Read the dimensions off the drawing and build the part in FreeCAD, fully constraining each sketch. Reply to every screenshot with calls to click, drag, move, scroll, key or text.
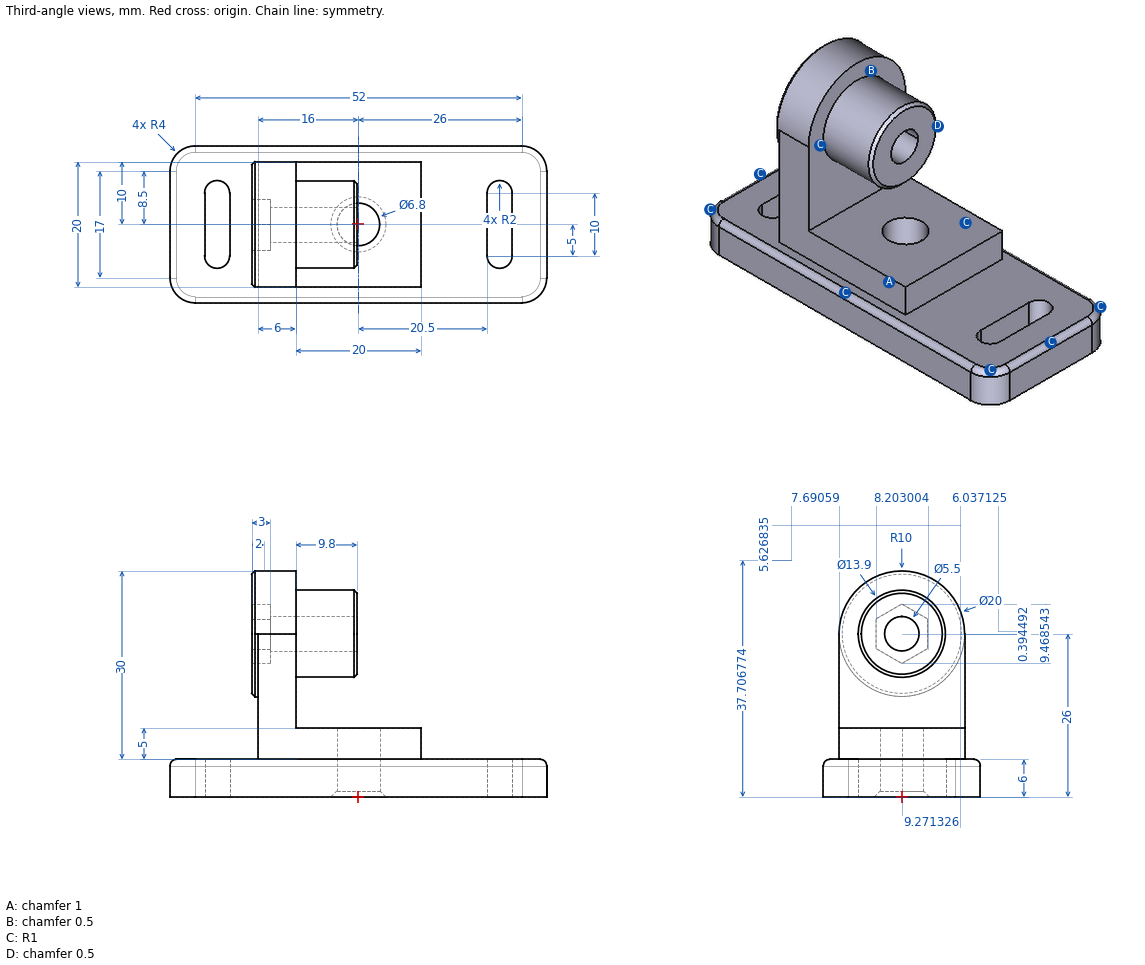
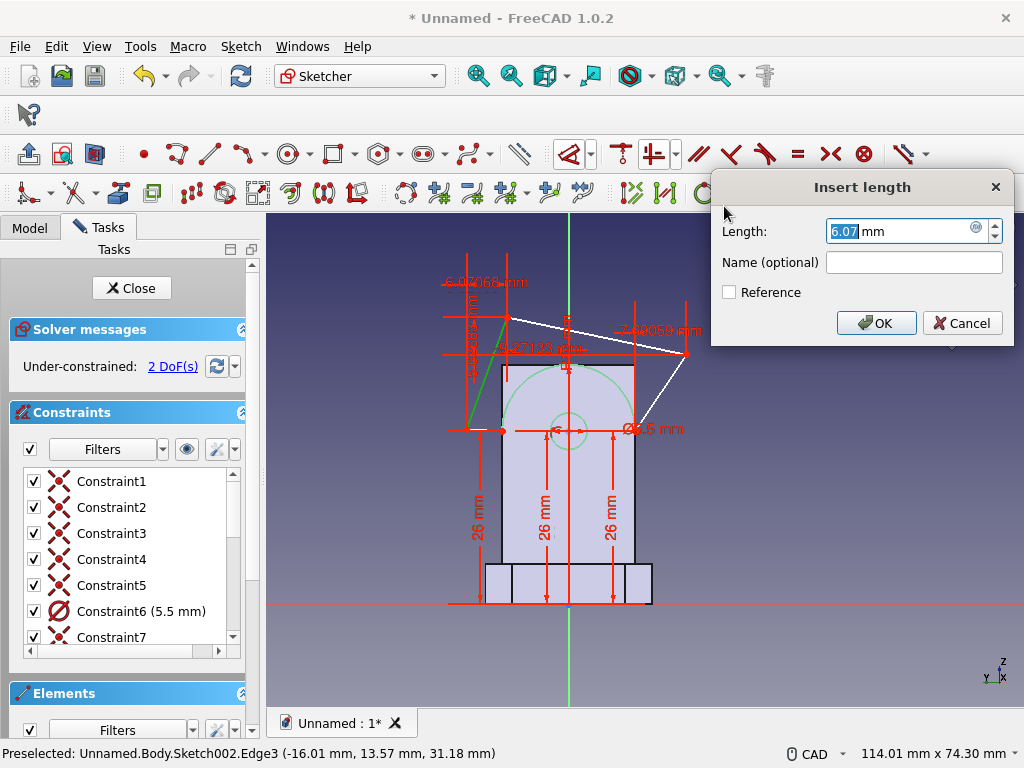
text(6.037125)
key(Return)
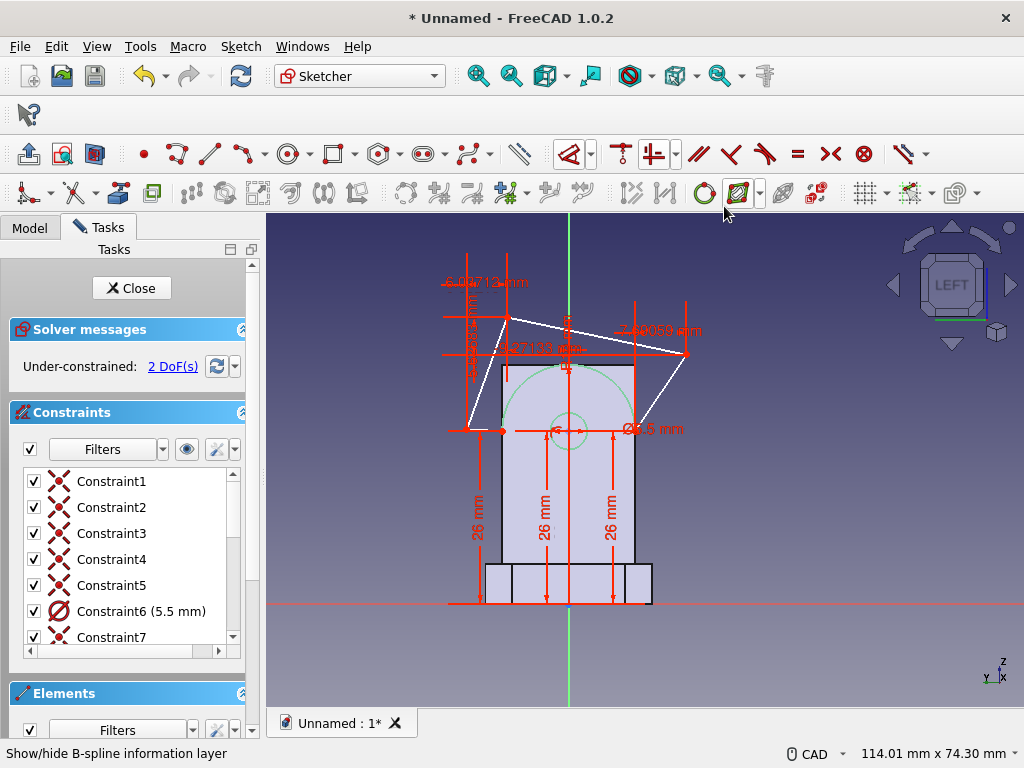
scroll(478, 430, up, 14)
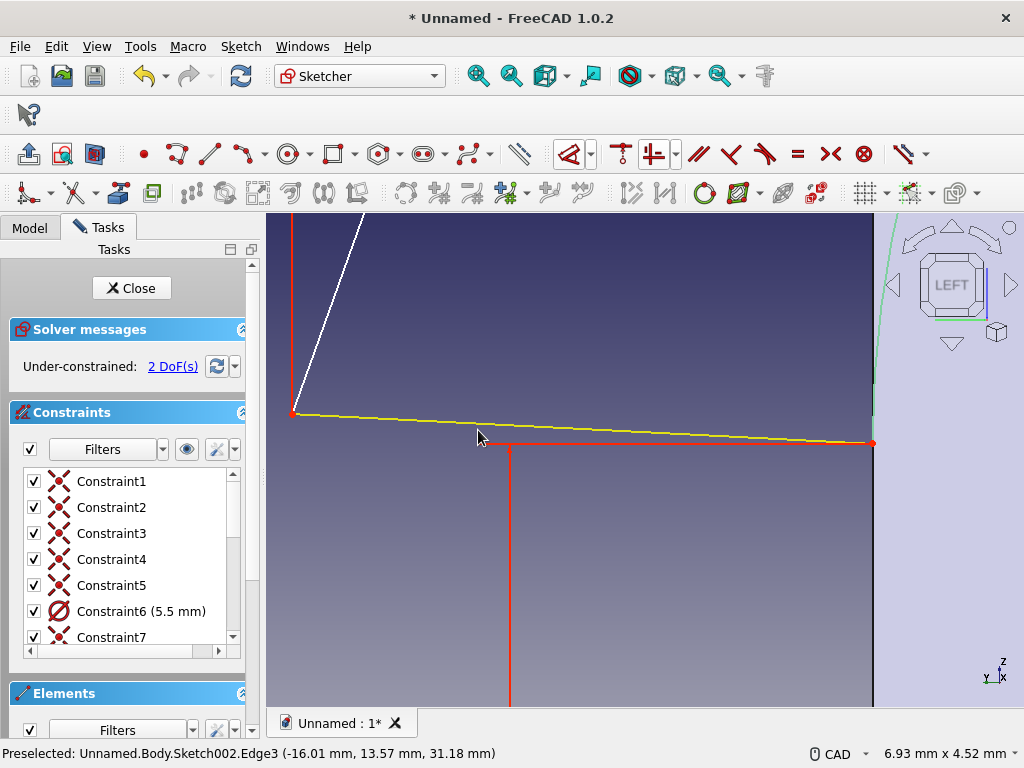
click(466, 423)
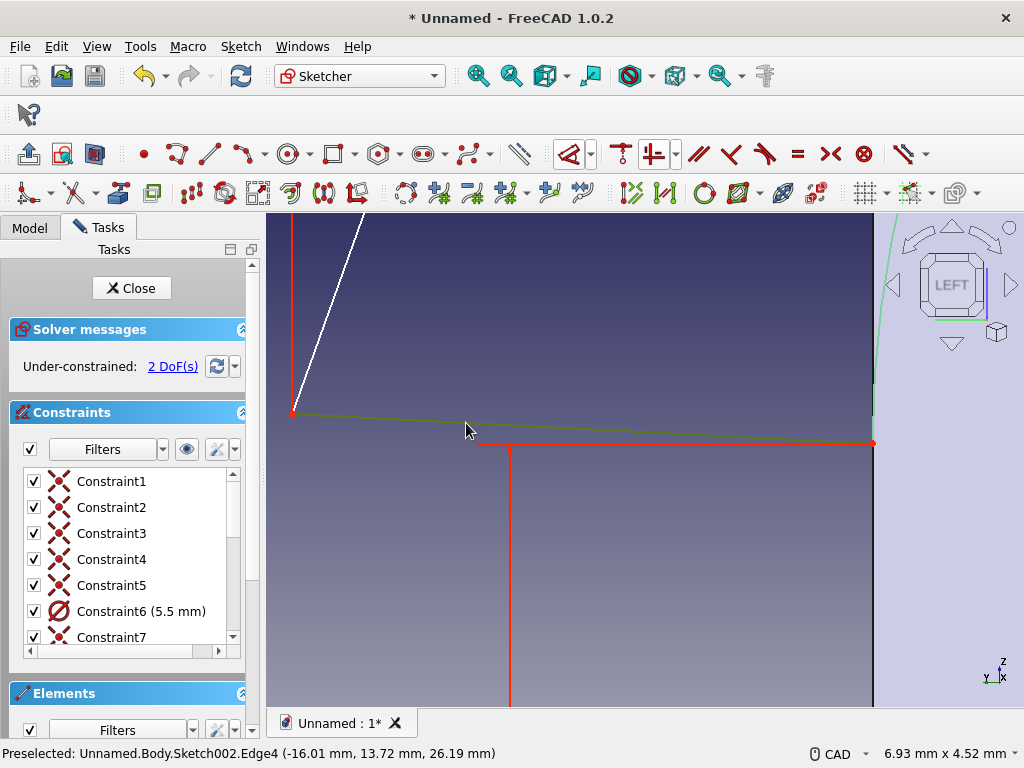
key(i)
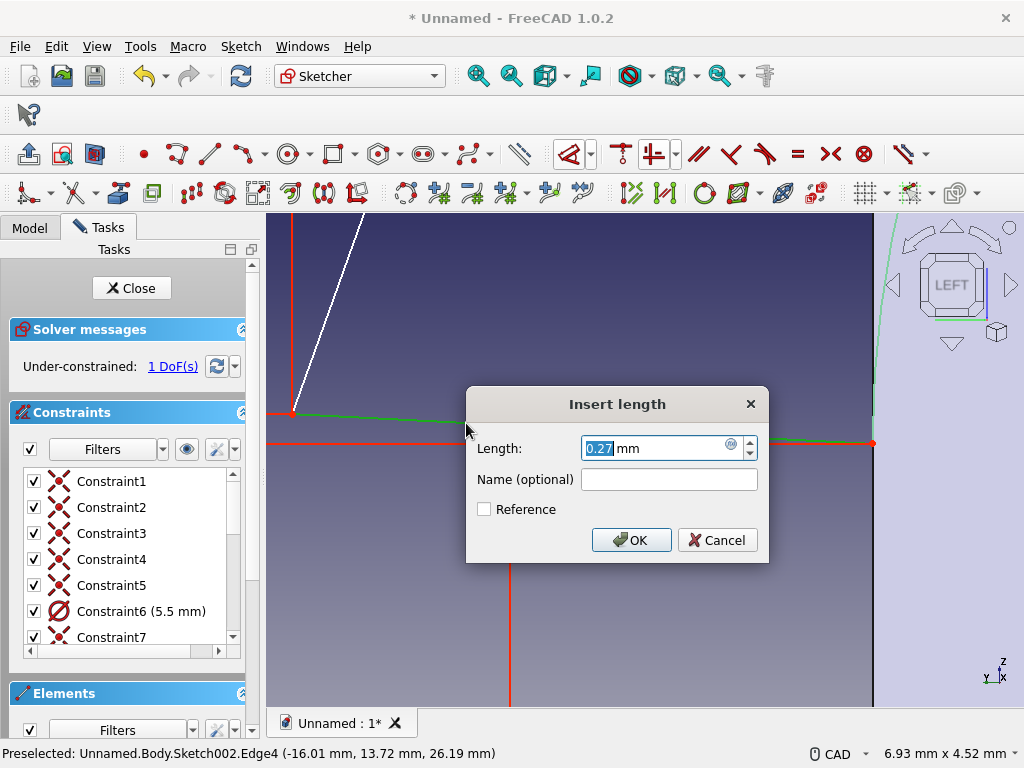
text(0.394492)
key(Return)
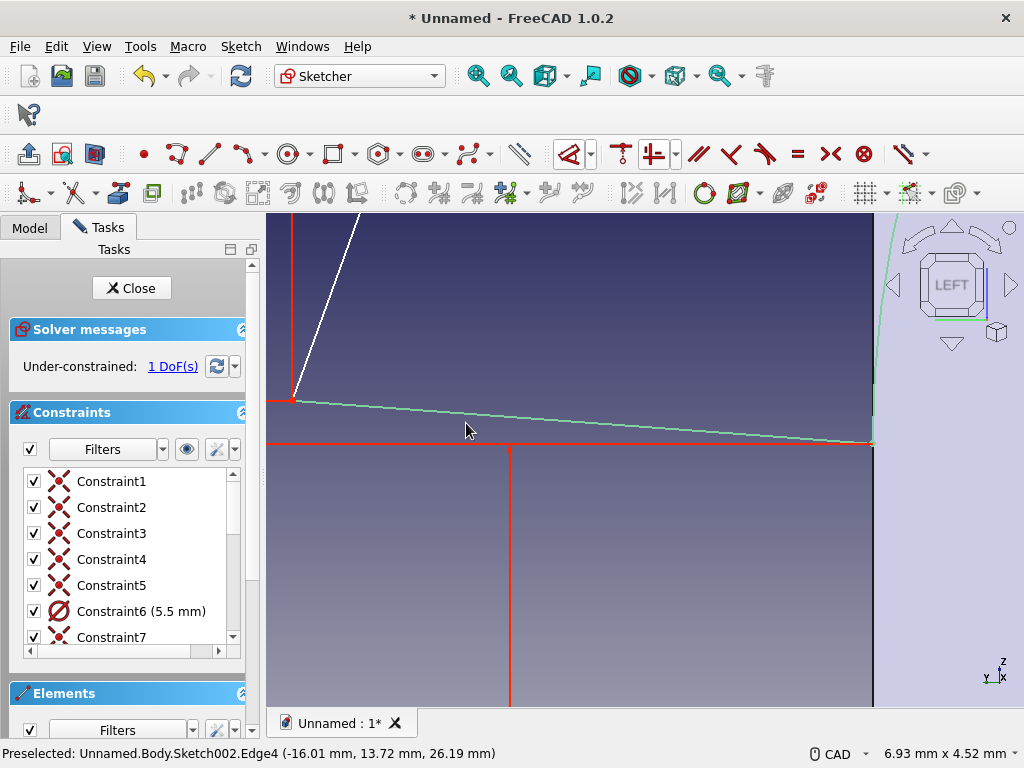
scroll(478, 430, down, 14)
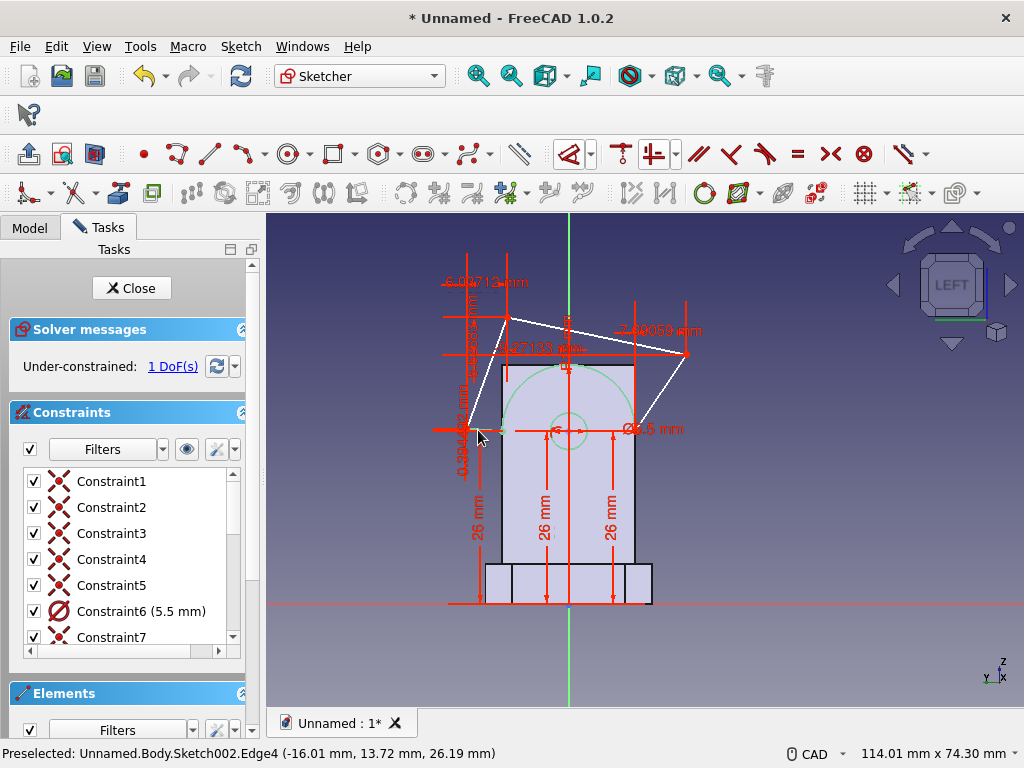
click(686, 355)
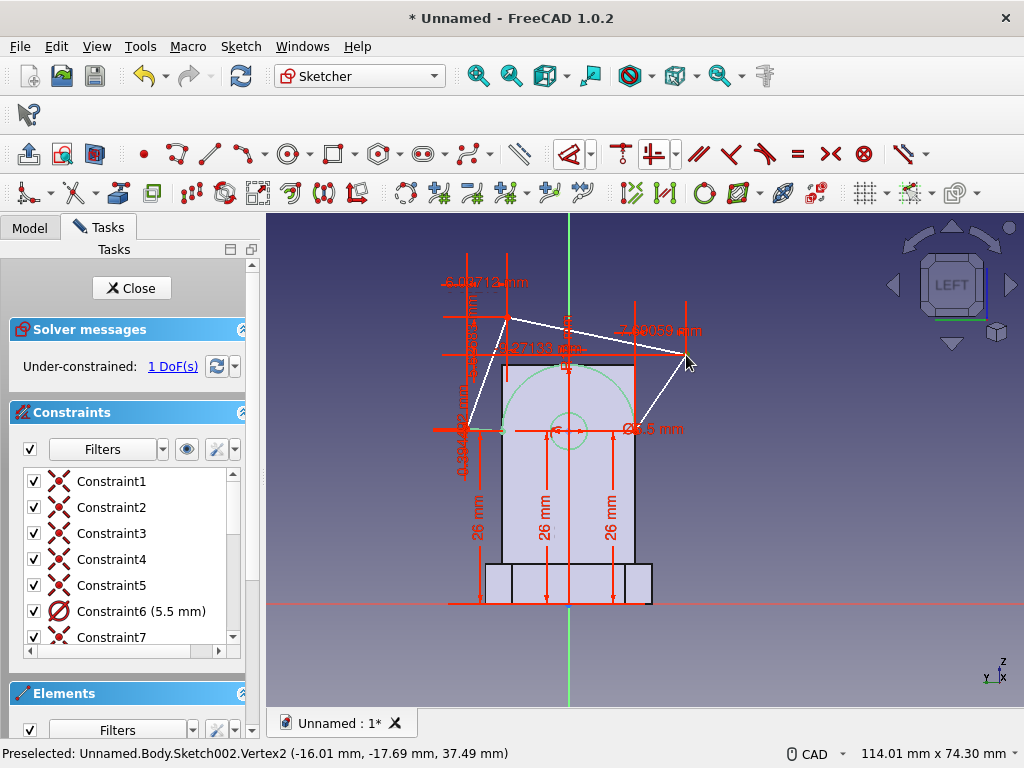
key(i)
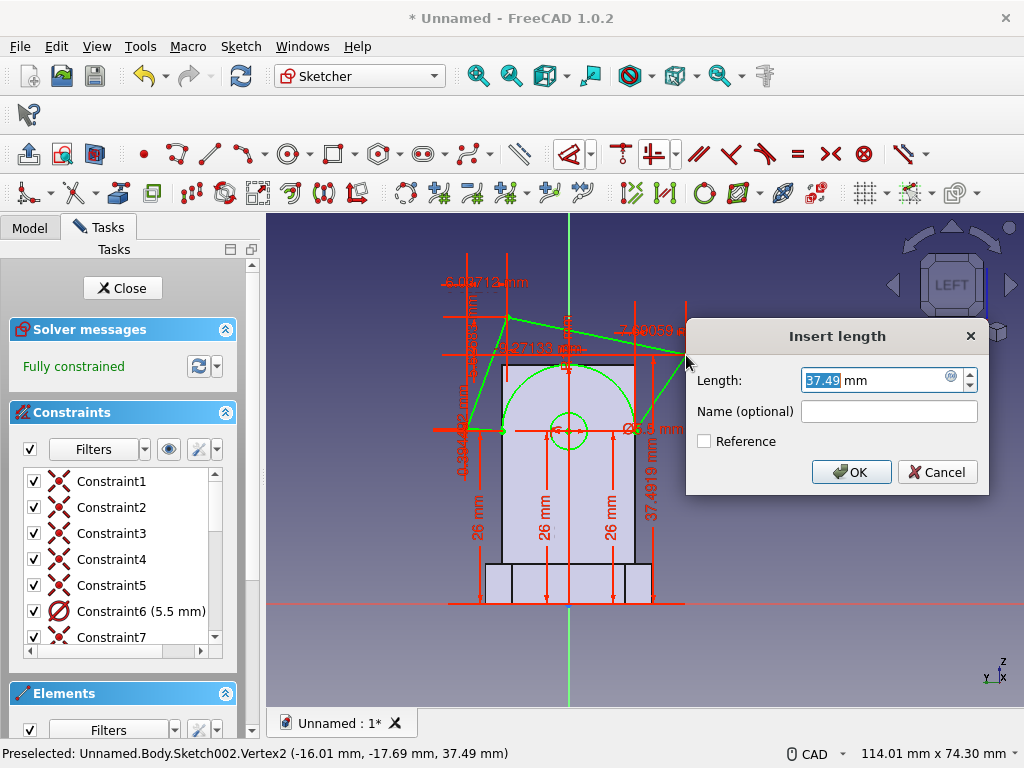
text(37.706774)
key(Return)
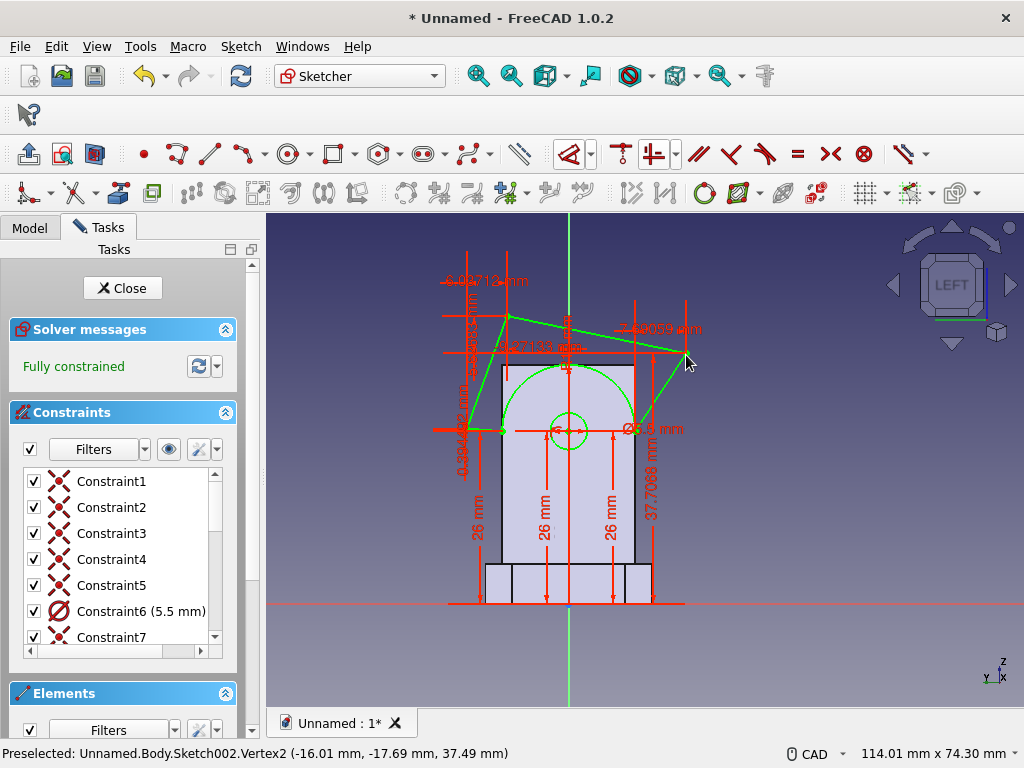
click(123, 288)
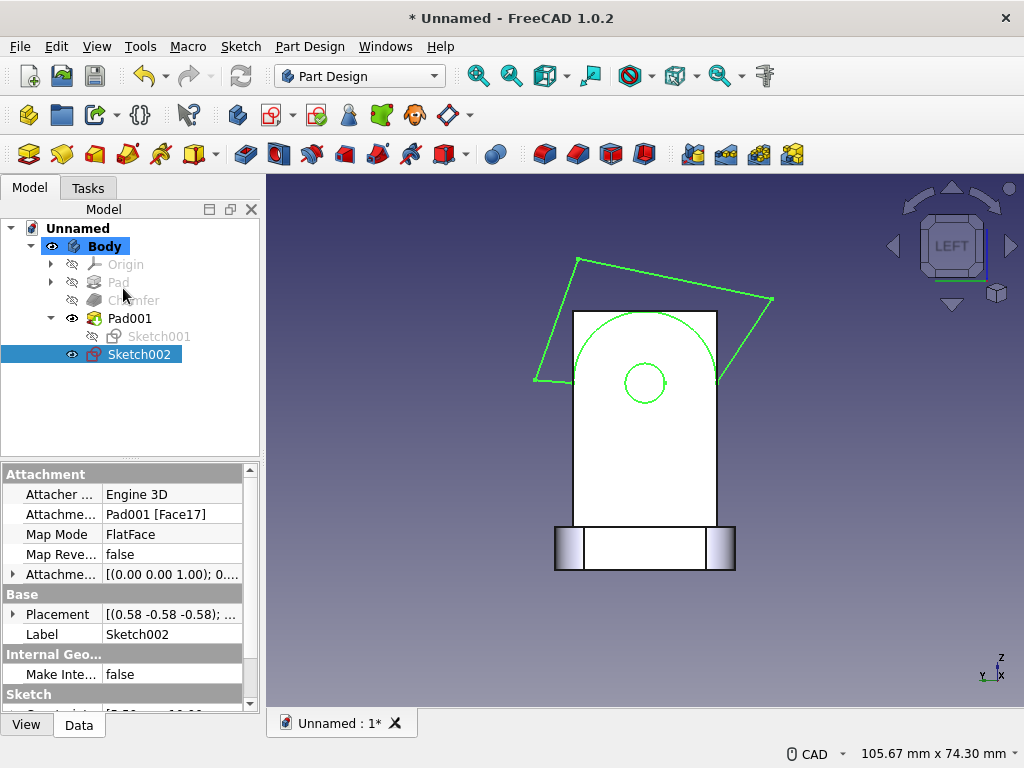
click(246, 154)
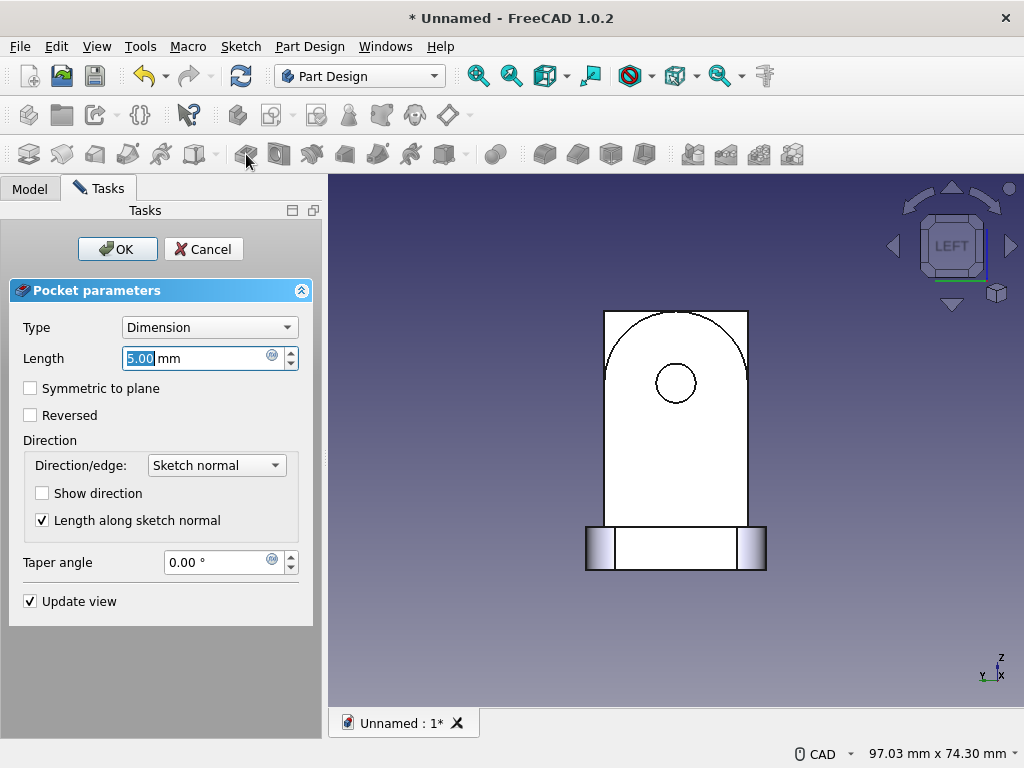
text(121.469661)
key(Tab)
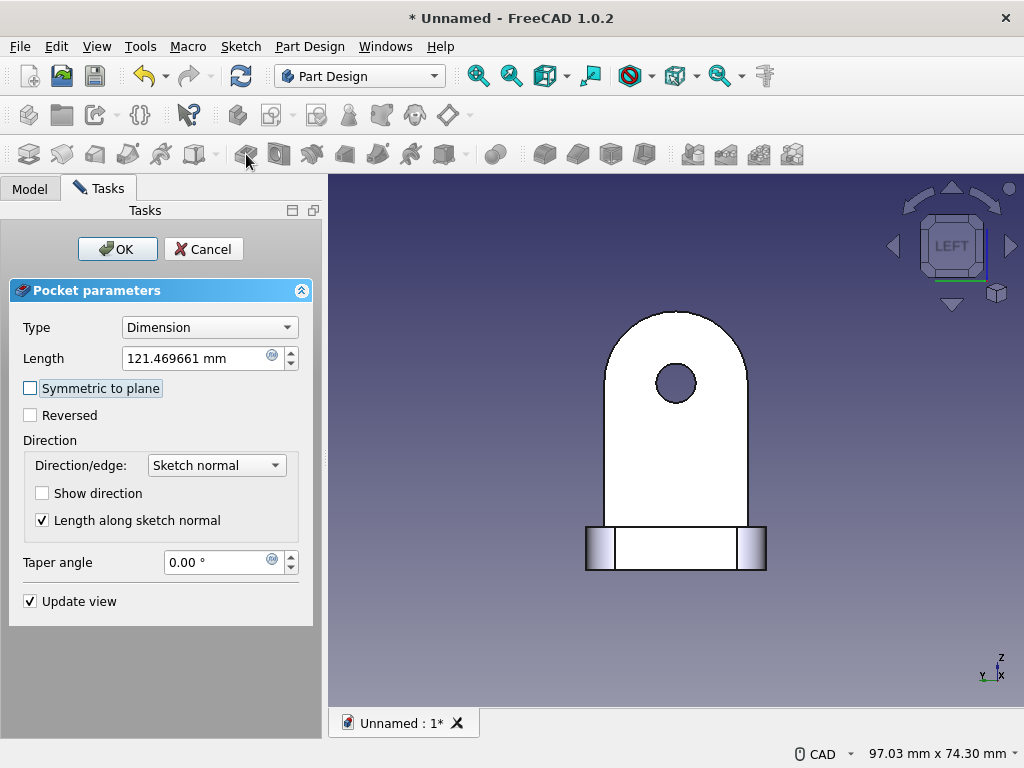
click(31, 388)